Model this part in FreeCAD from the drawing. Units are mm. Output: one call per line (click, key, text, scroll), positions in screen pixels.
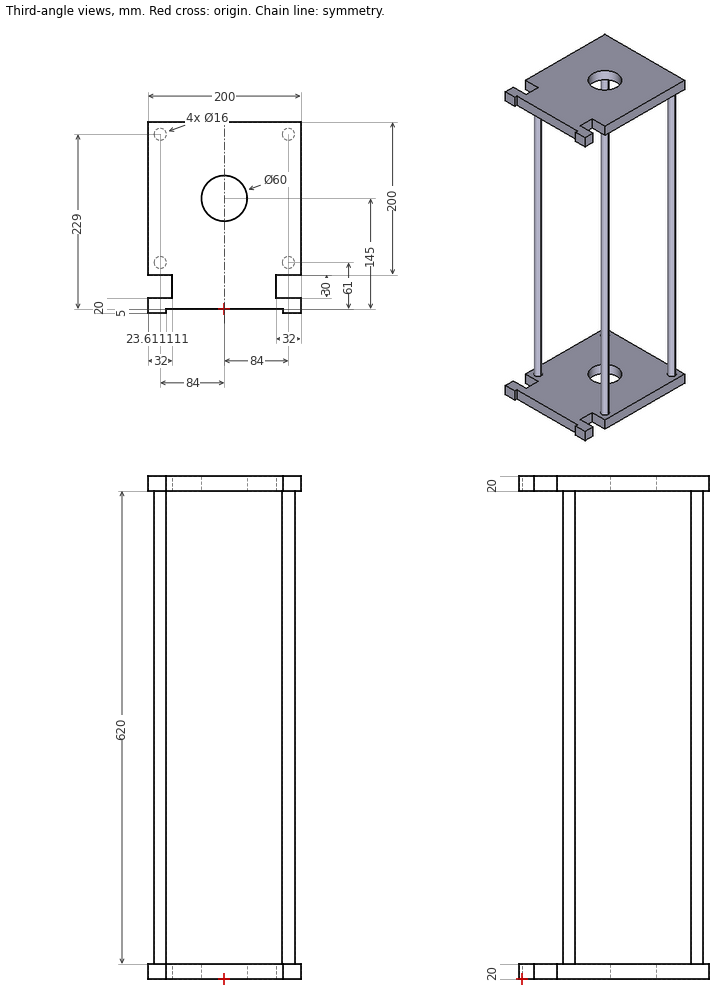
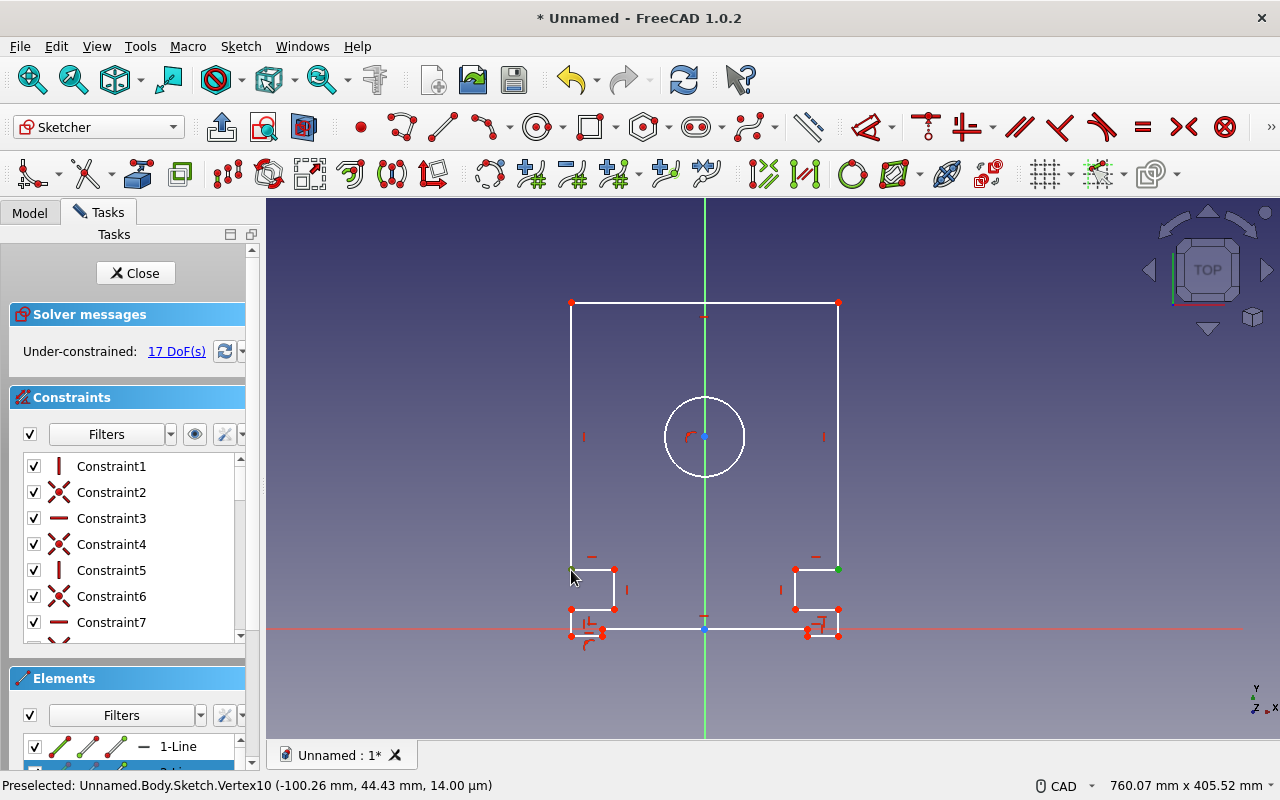
click(705, 676)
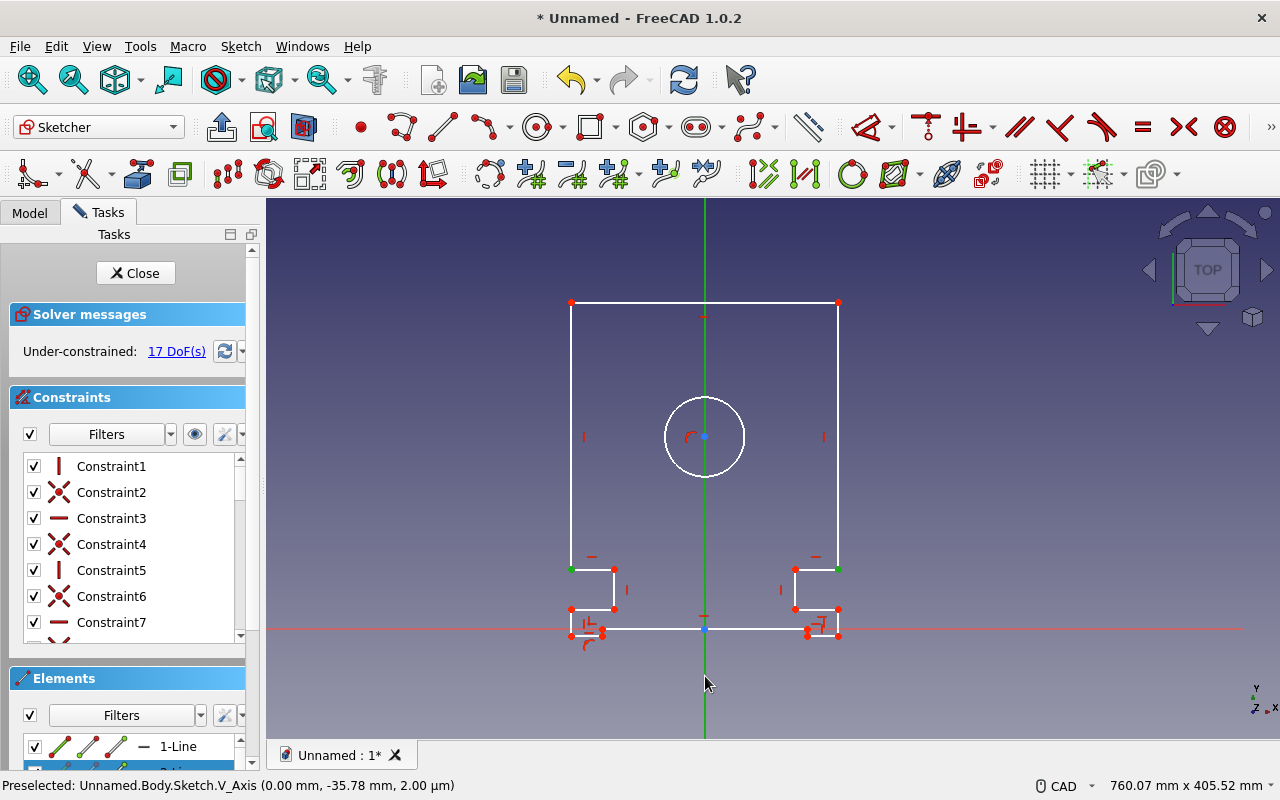
click(1184, 128)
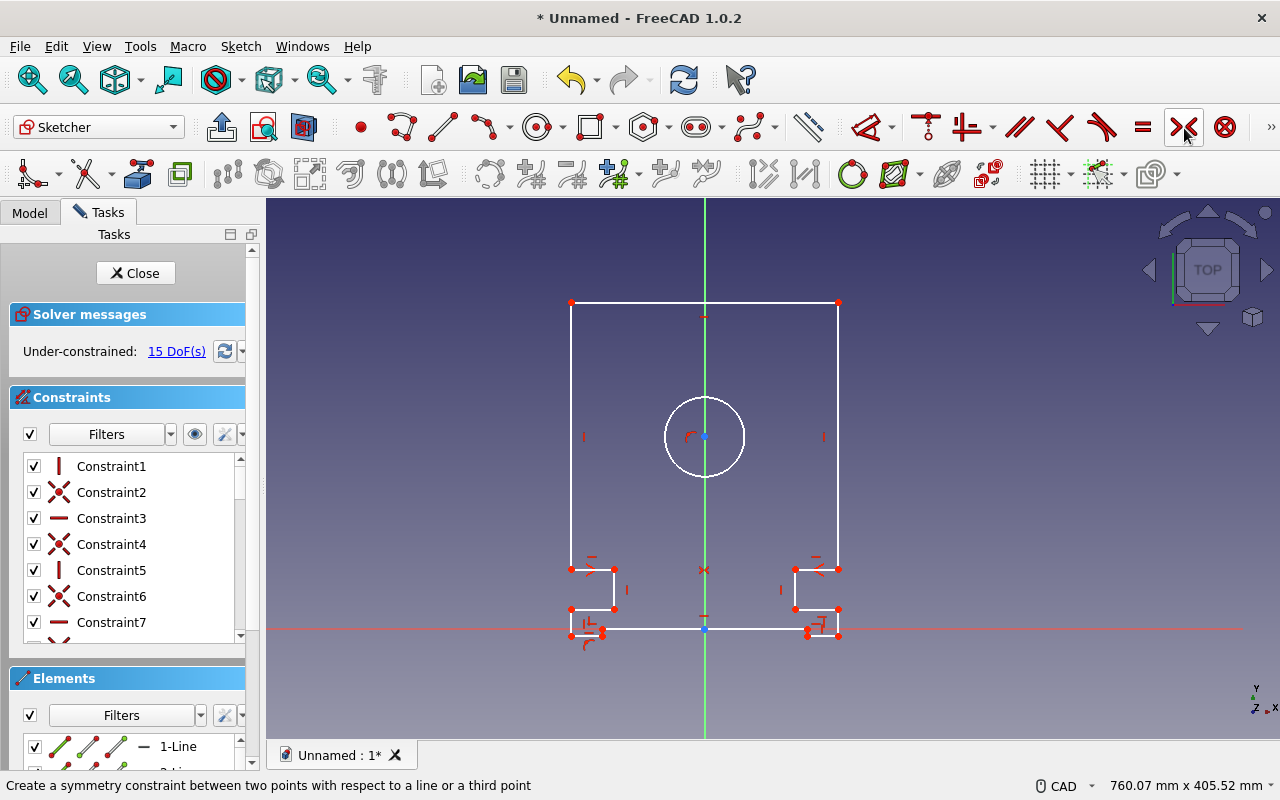
click(795, 610)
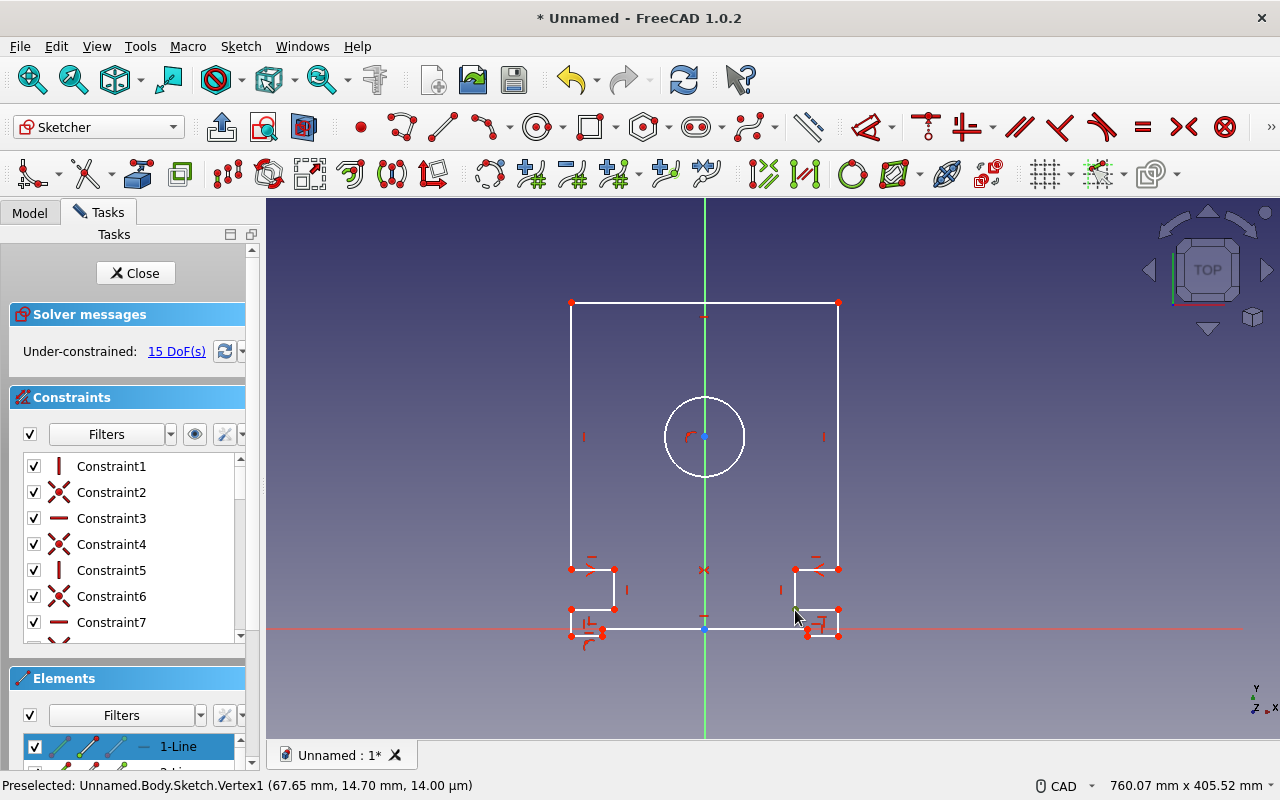
click(614, 610)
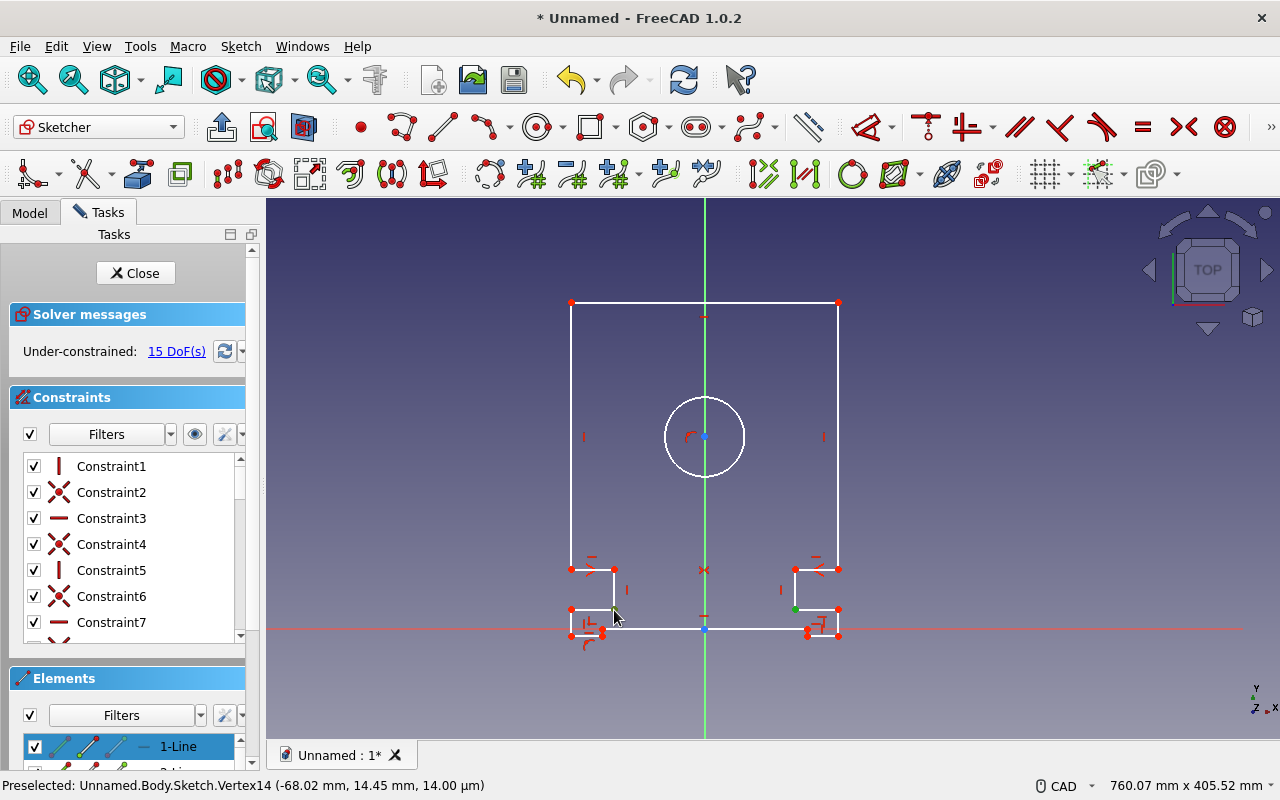
click(705, 676)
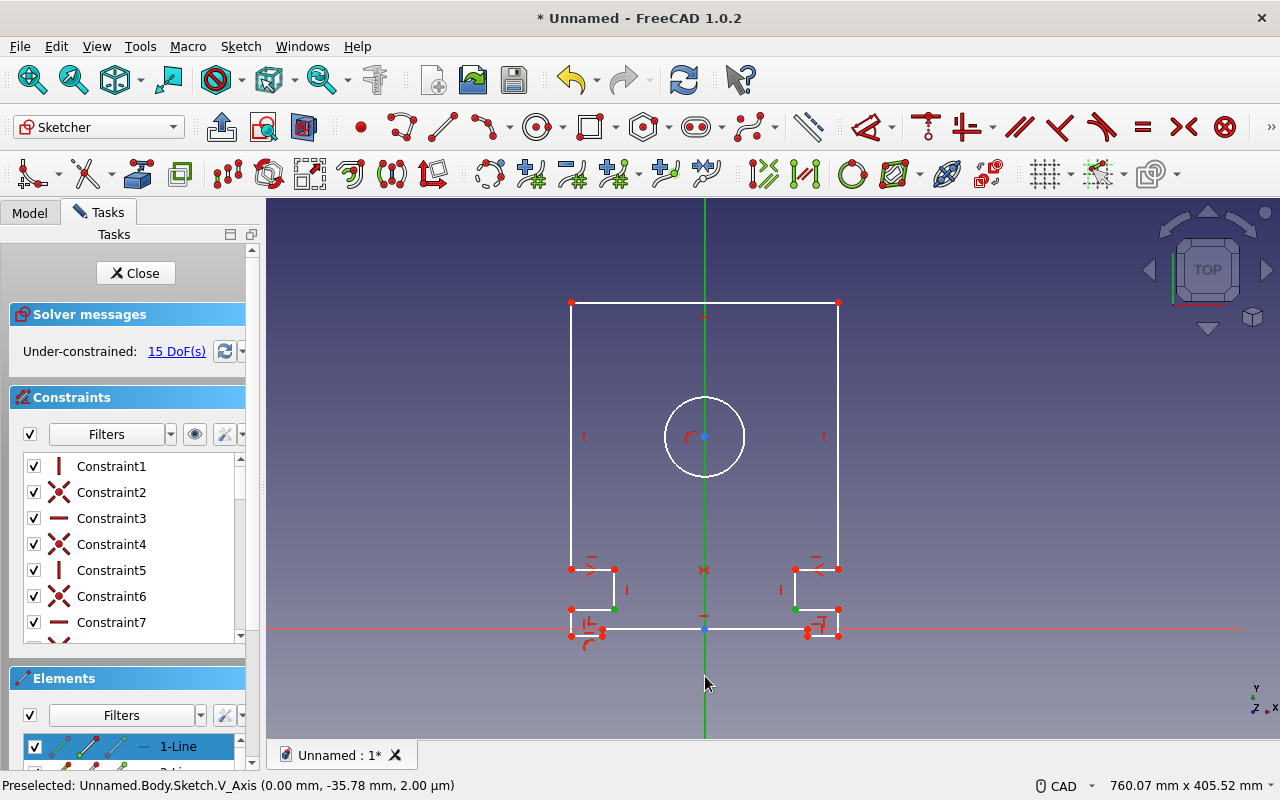
click(1184, 128)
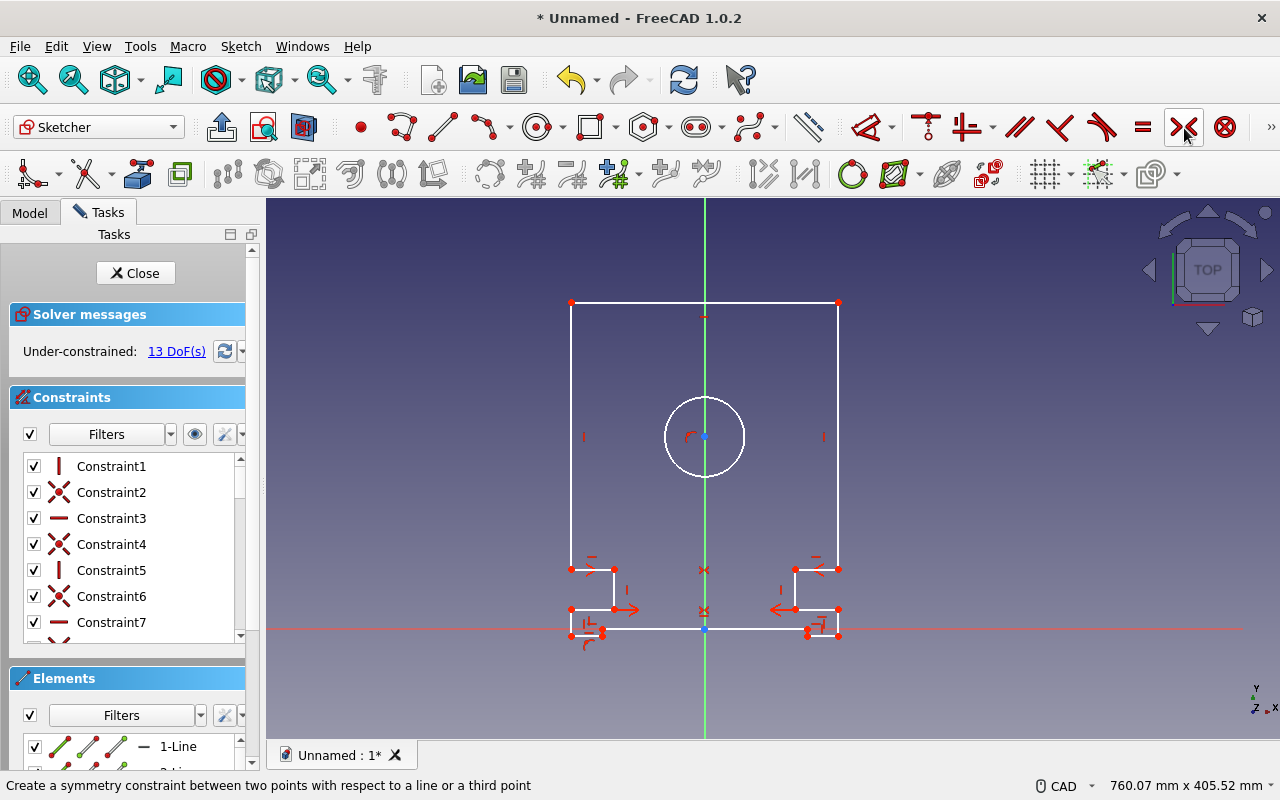
scroll(603, 636, up, 3)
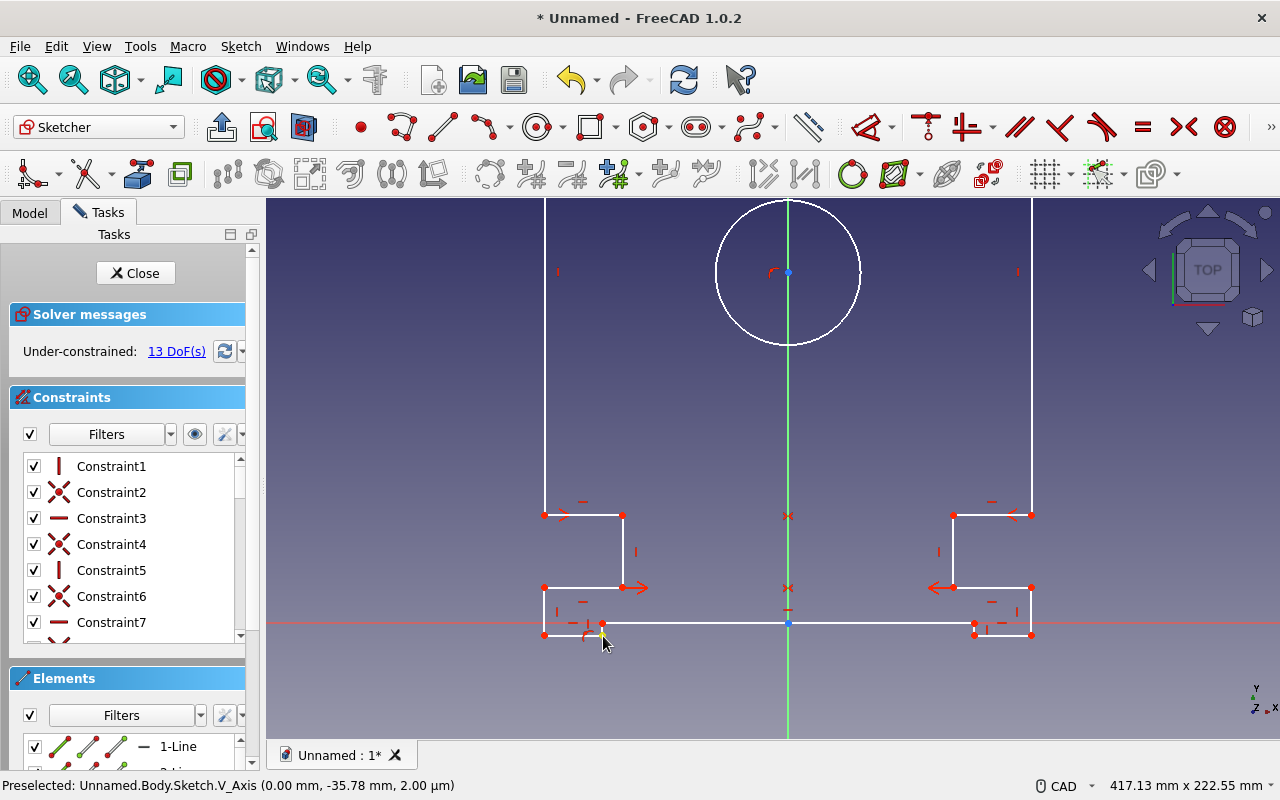
click(602, 636)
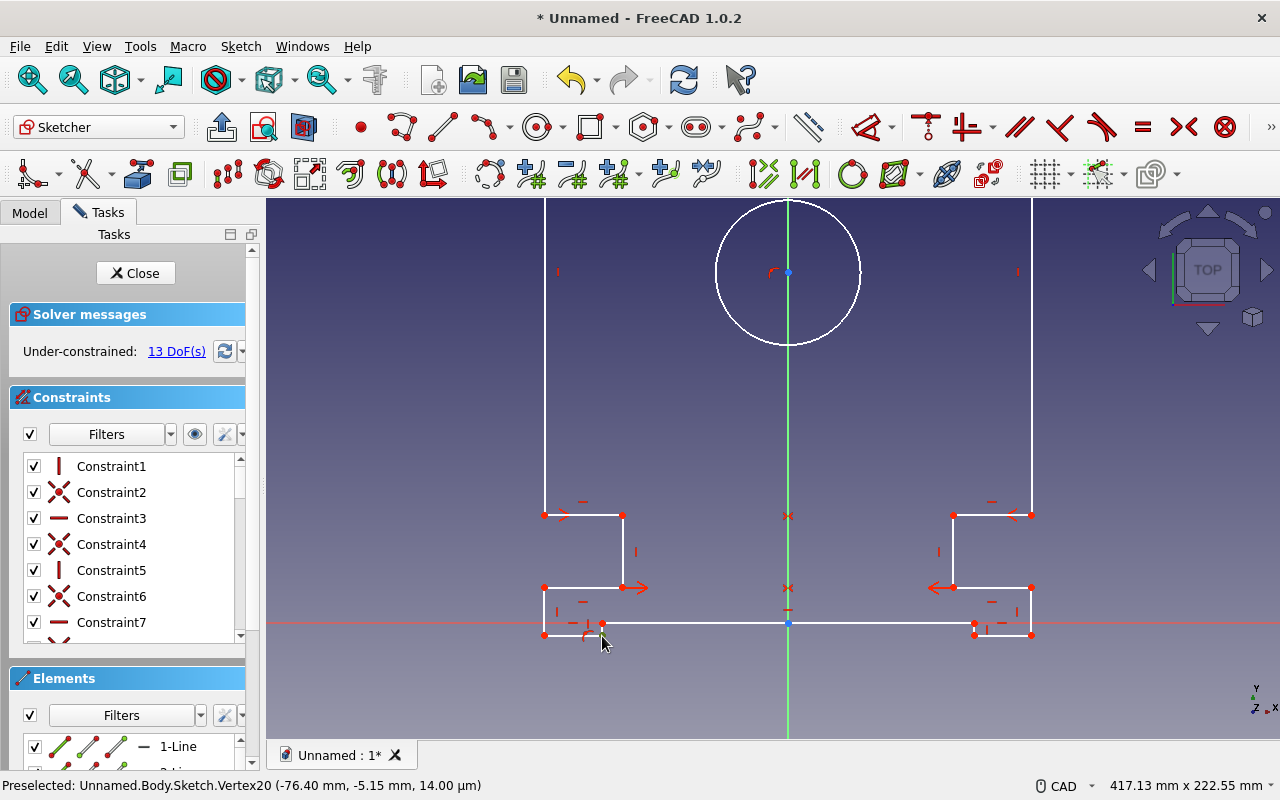
click(974, 636)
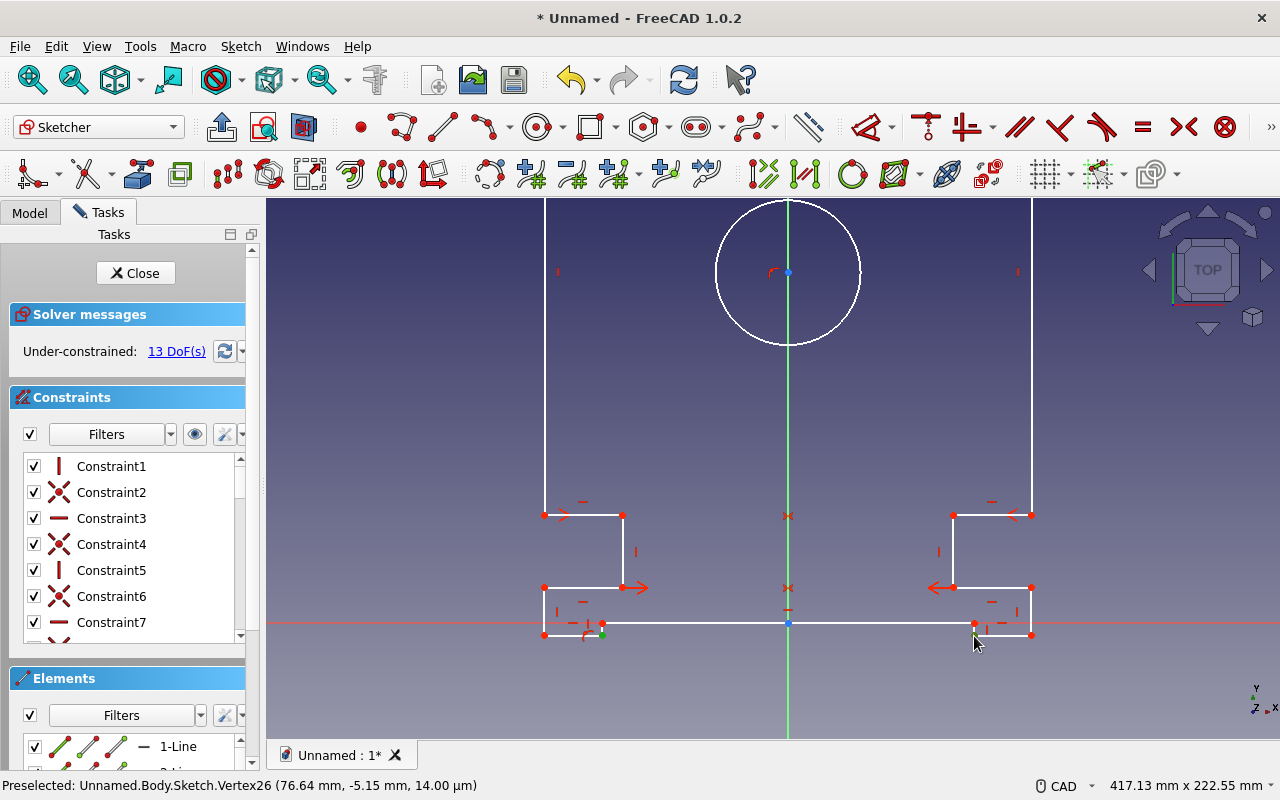
click(788, 676)